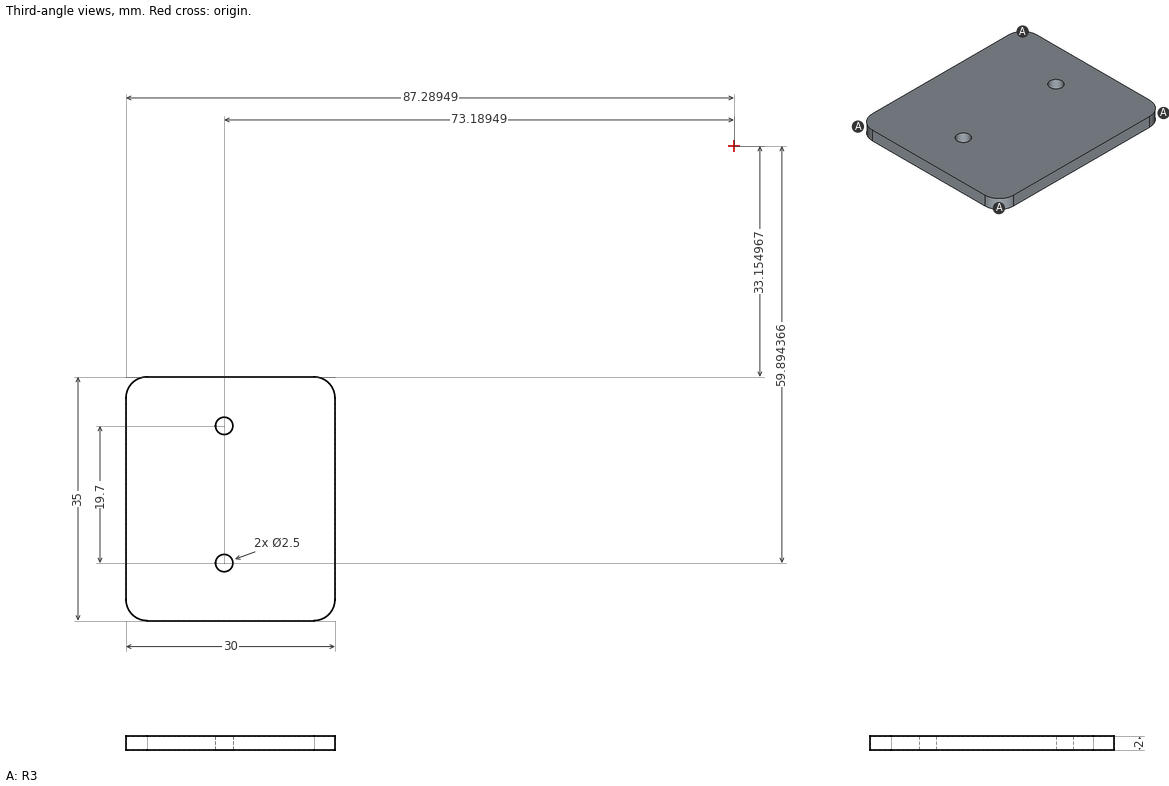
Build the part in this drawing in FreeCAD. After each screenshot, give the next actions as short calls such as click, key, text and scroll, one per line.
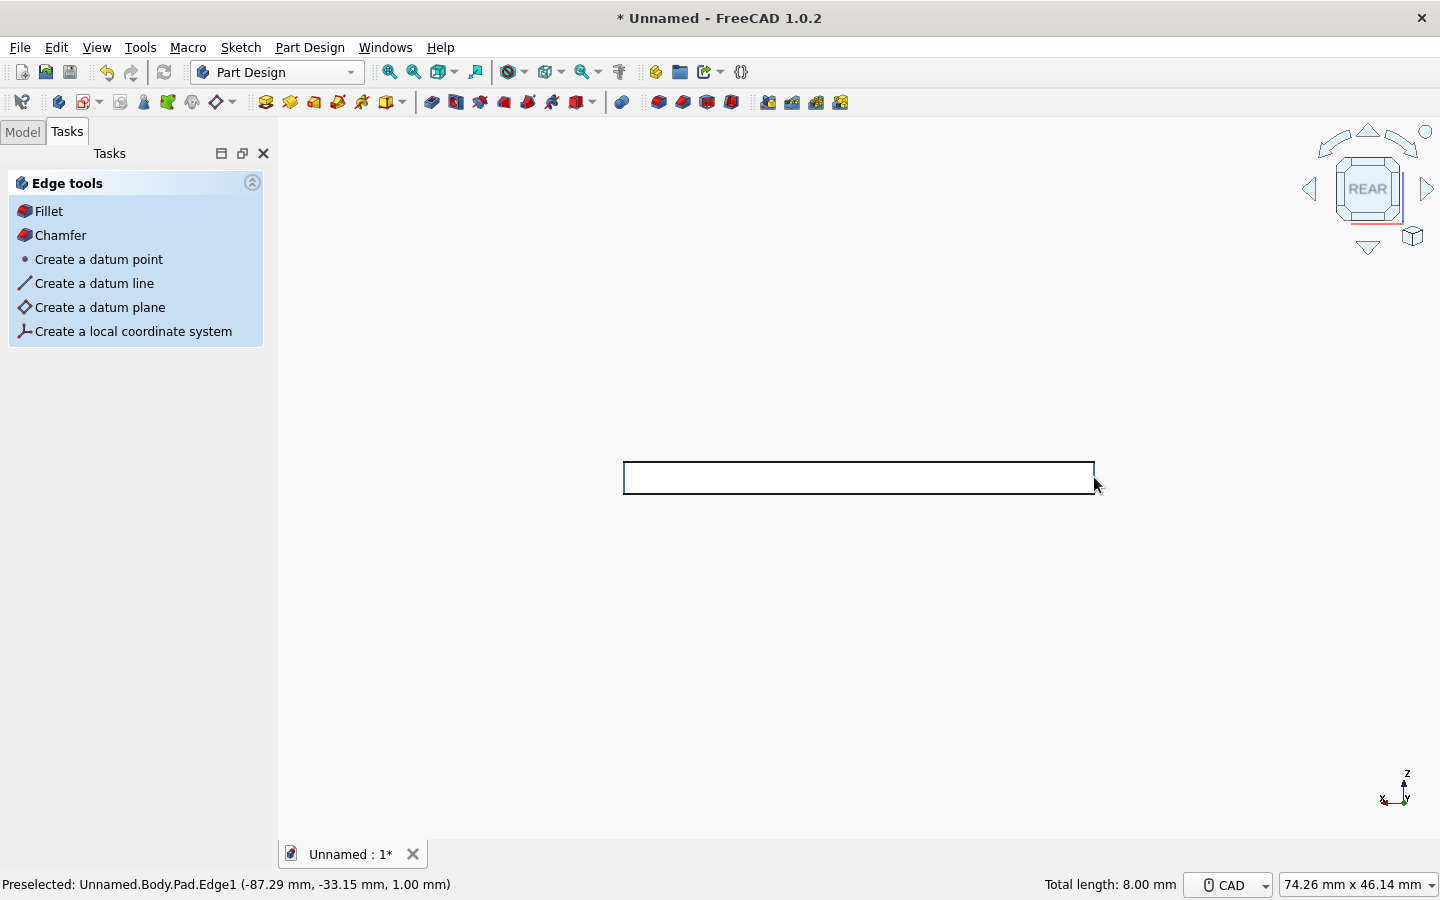
click(660, 102)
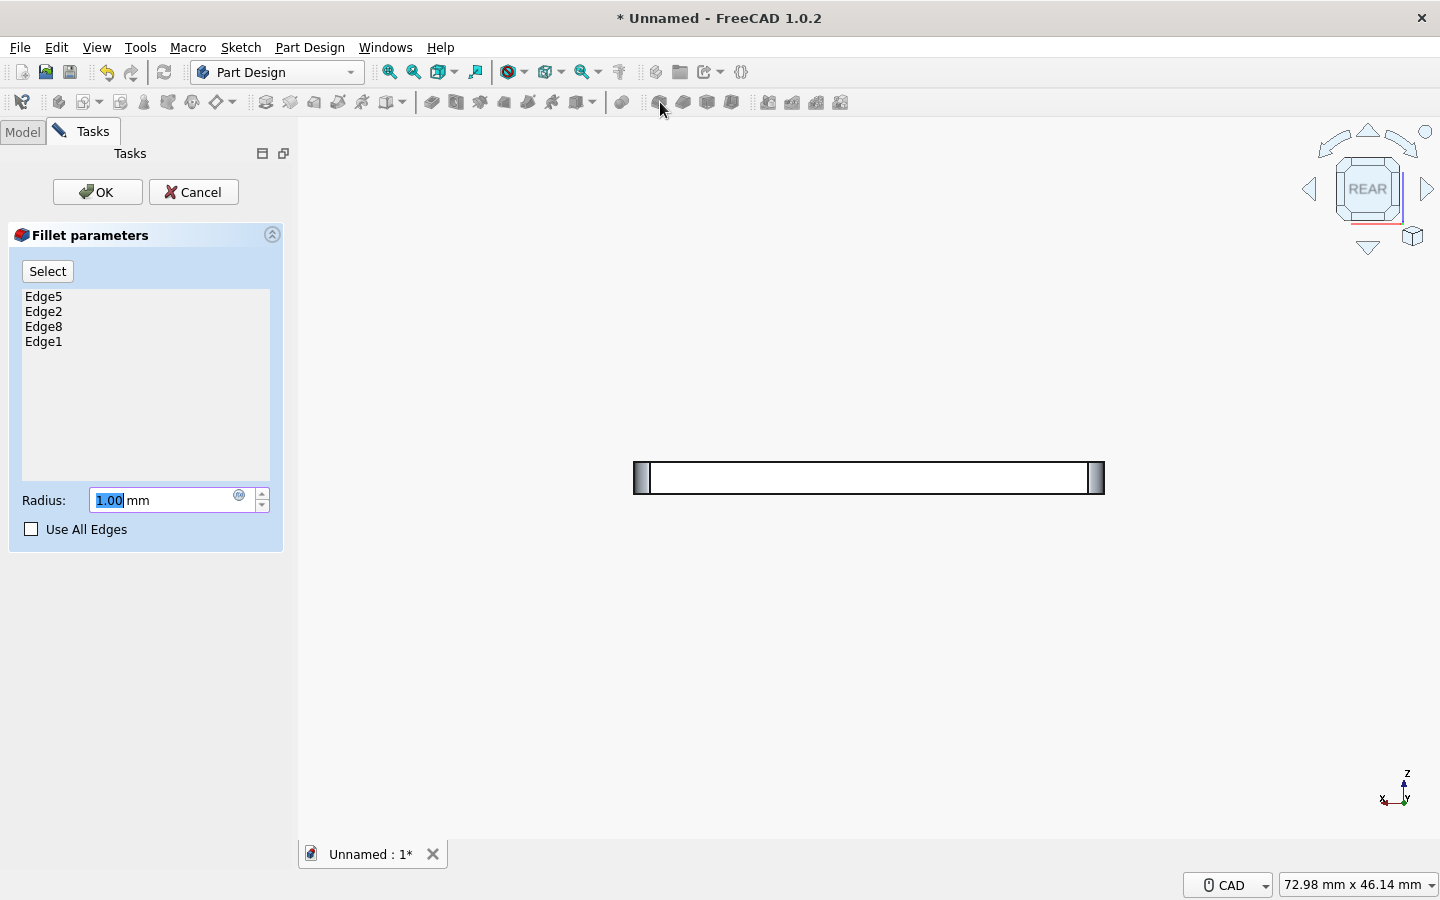
text(3)
key(Tab)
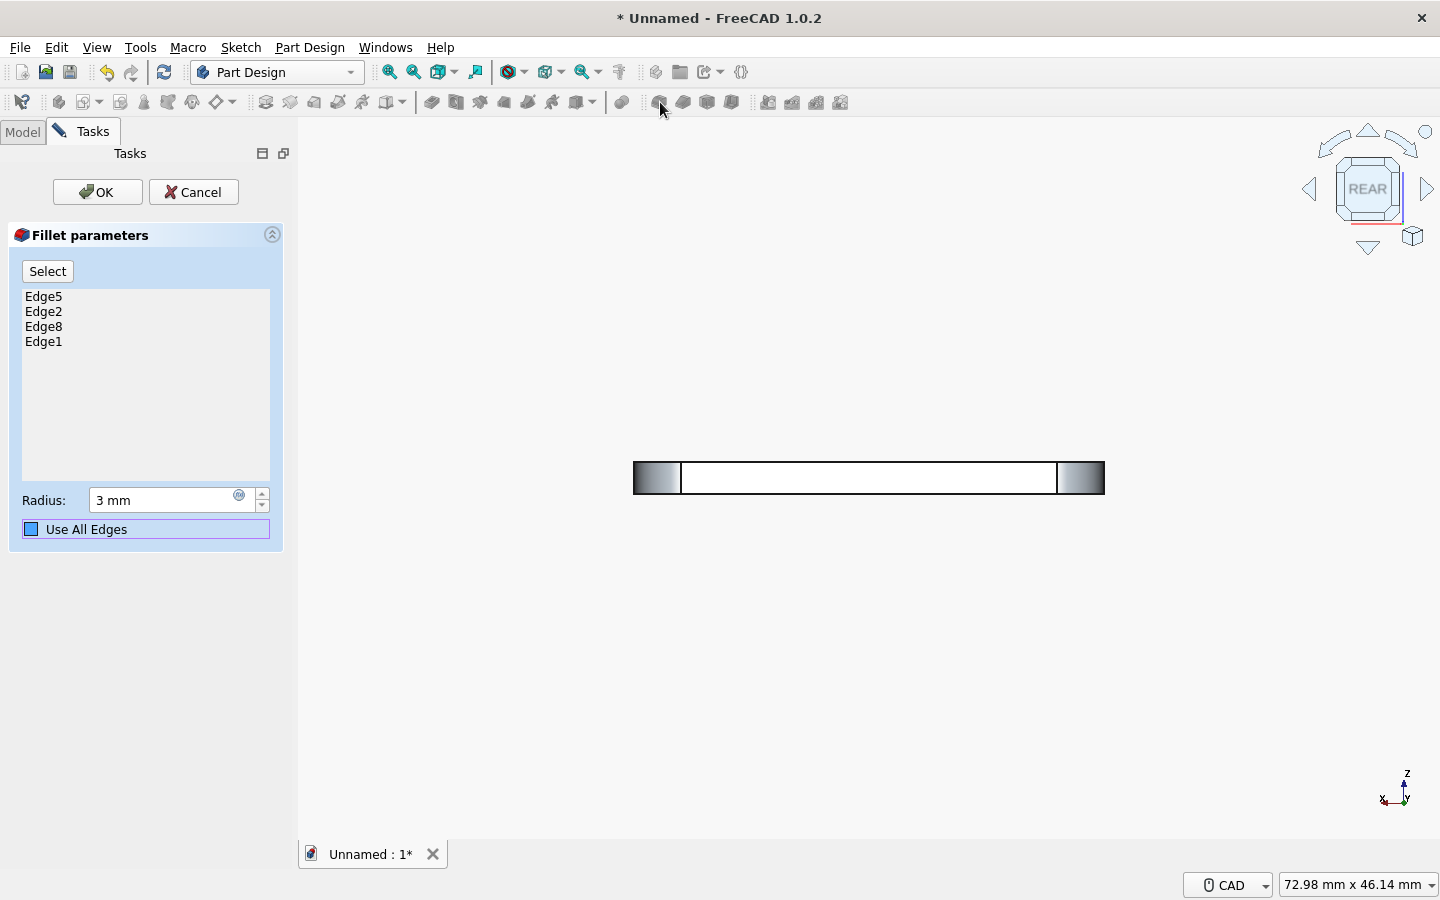
click(98, 192)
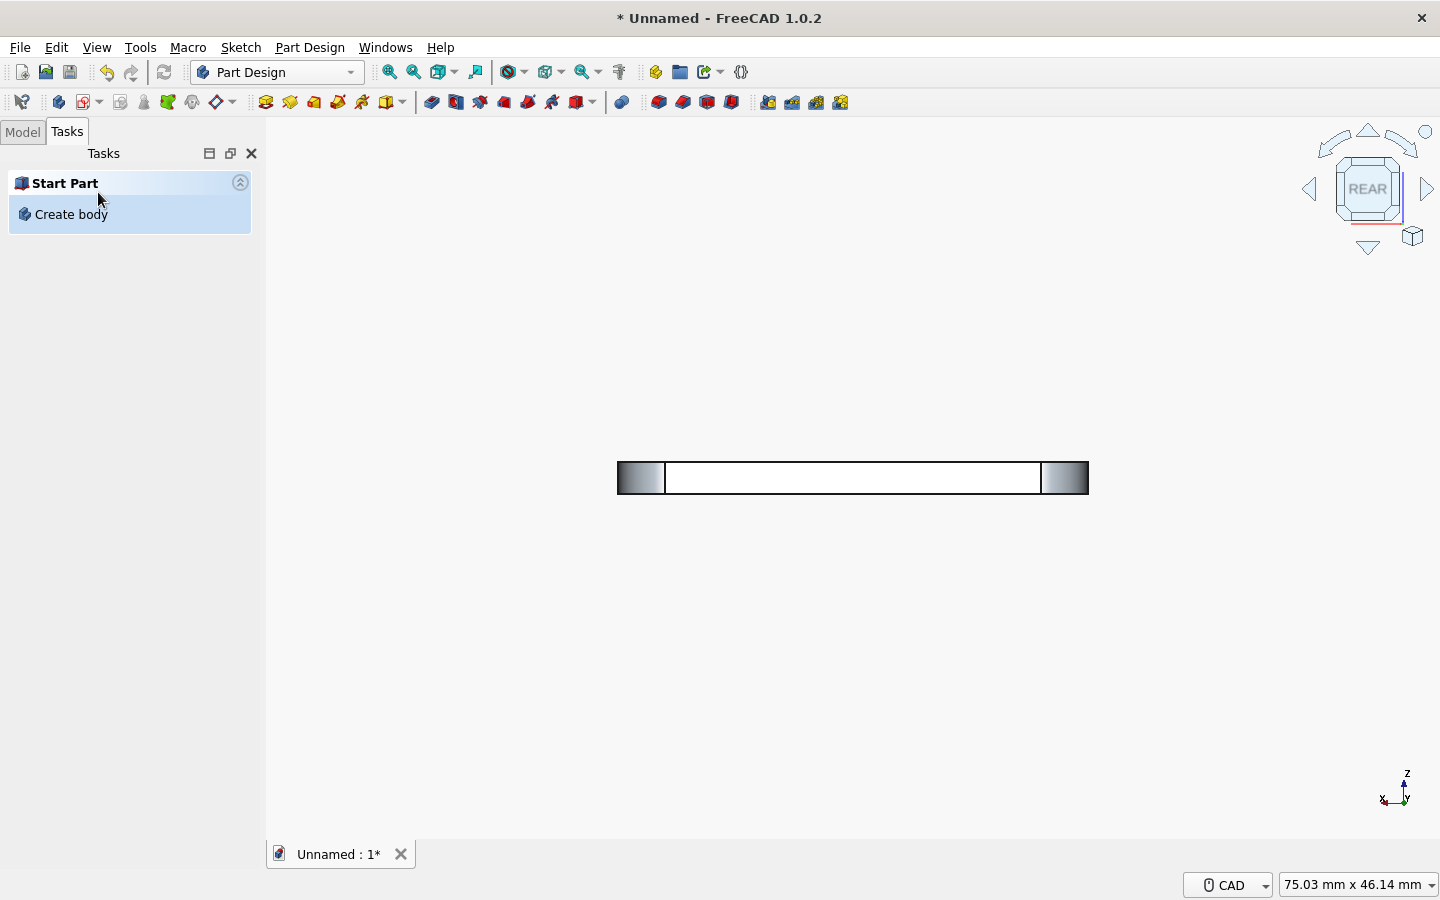
click(390, 72)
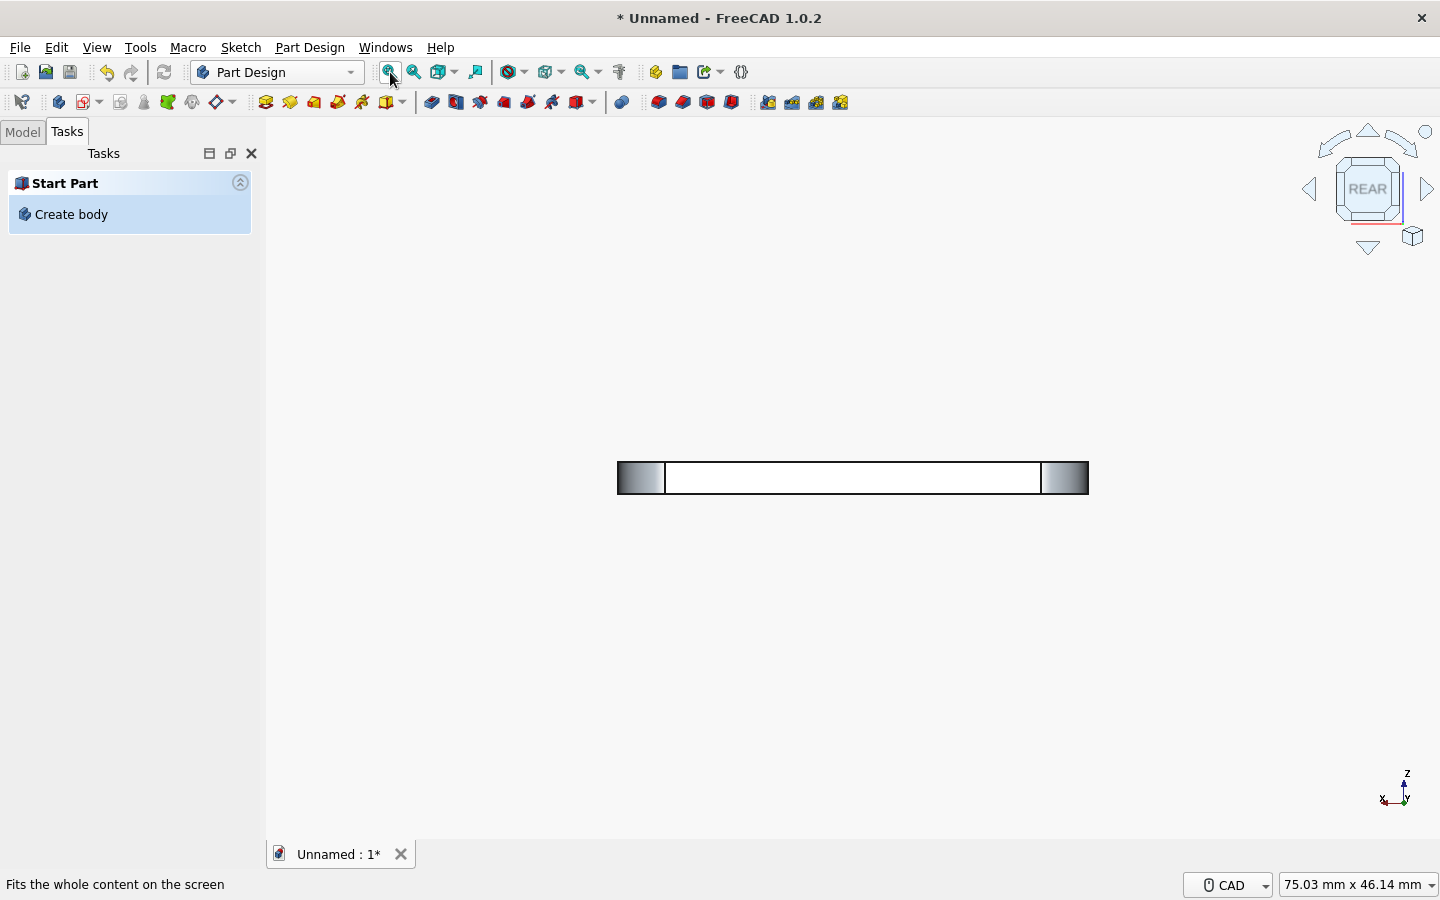
key(0)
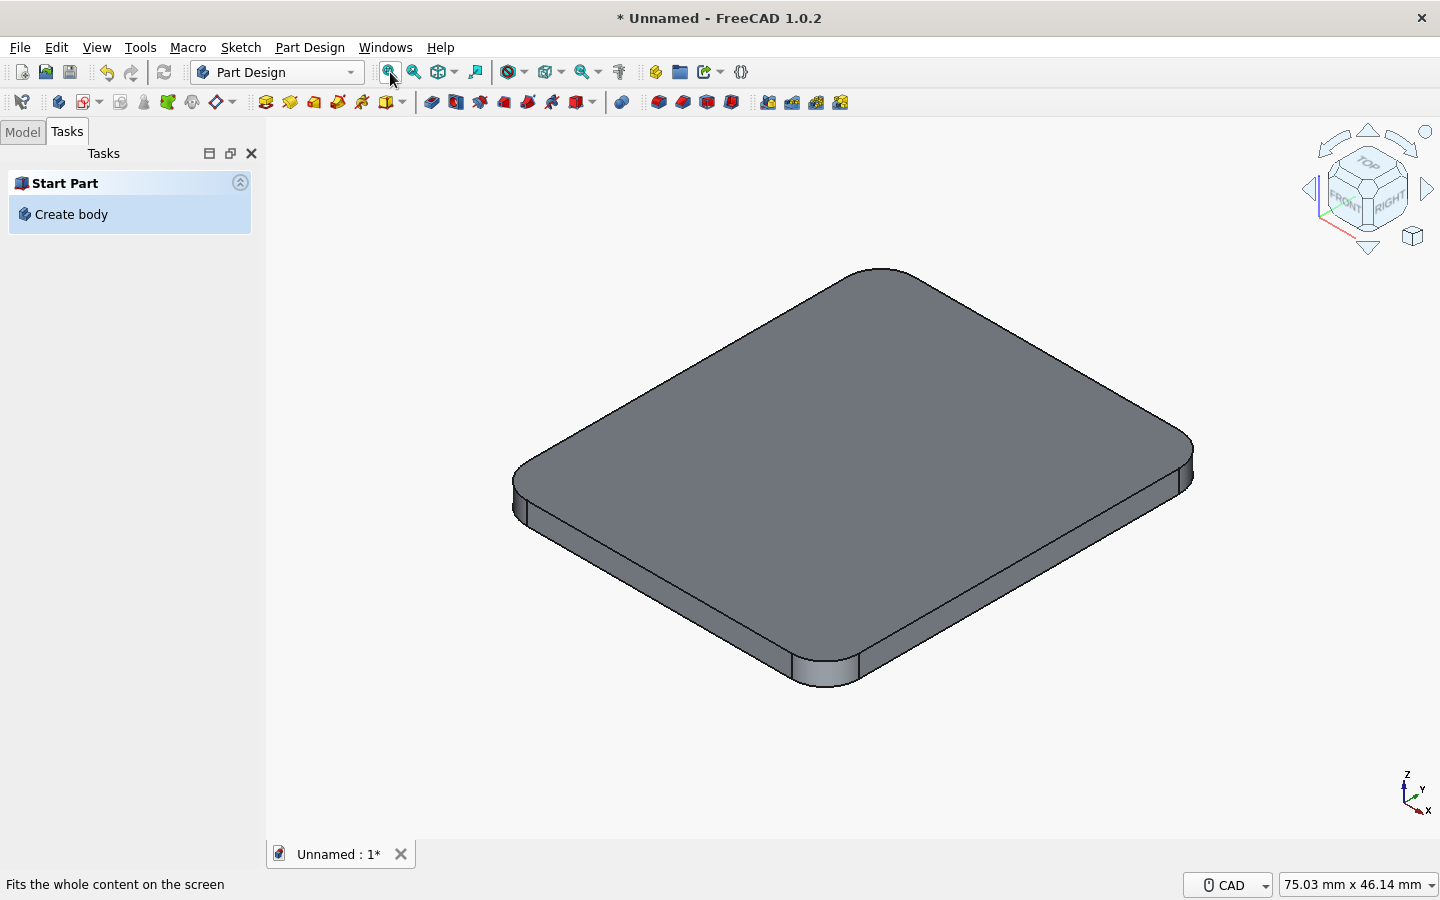
click(853, 464)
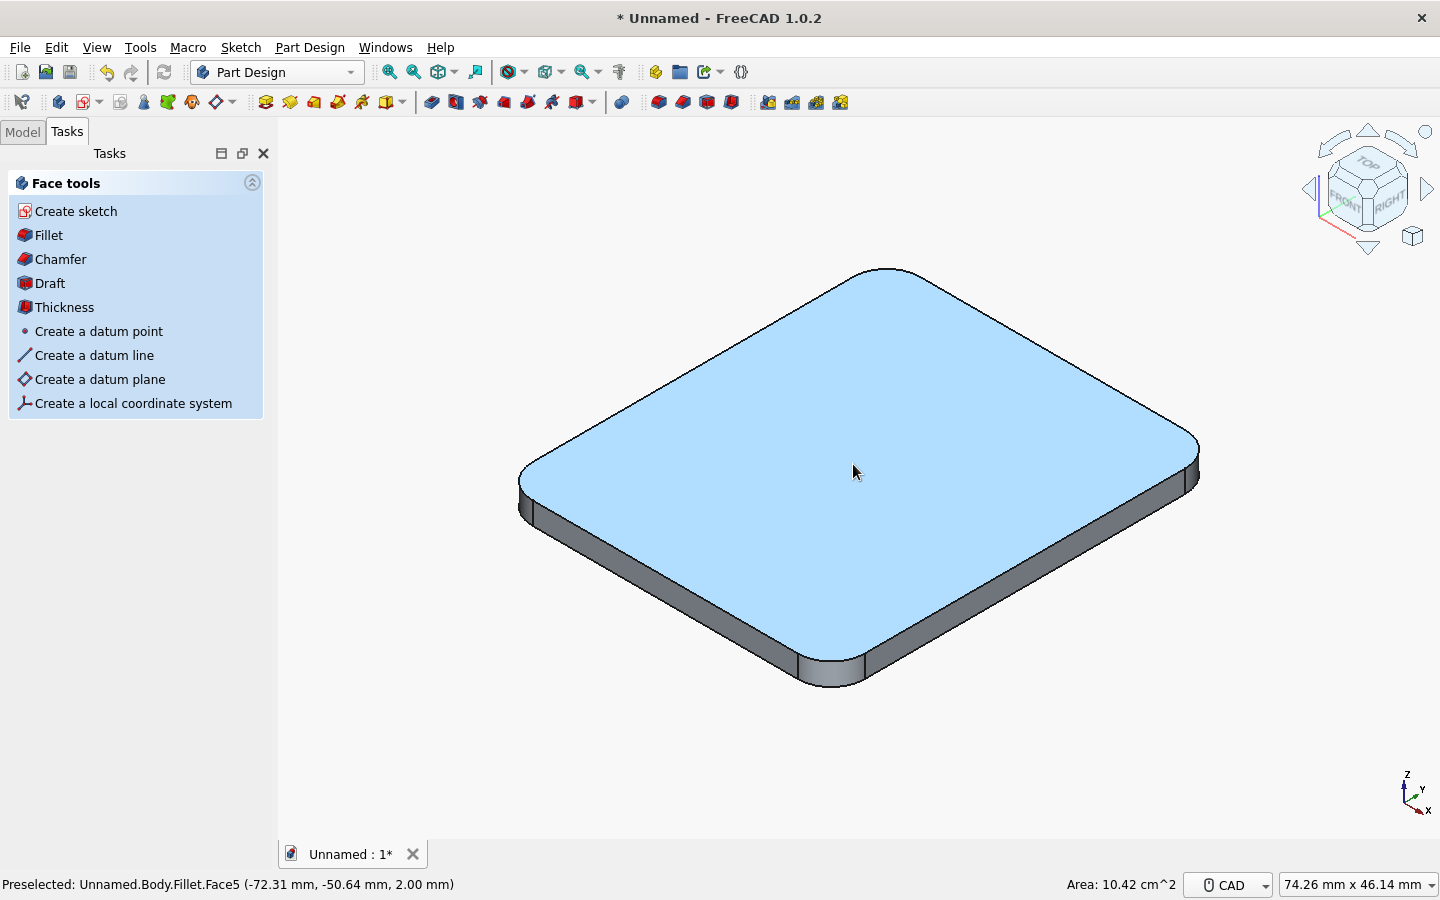
click(84, 102)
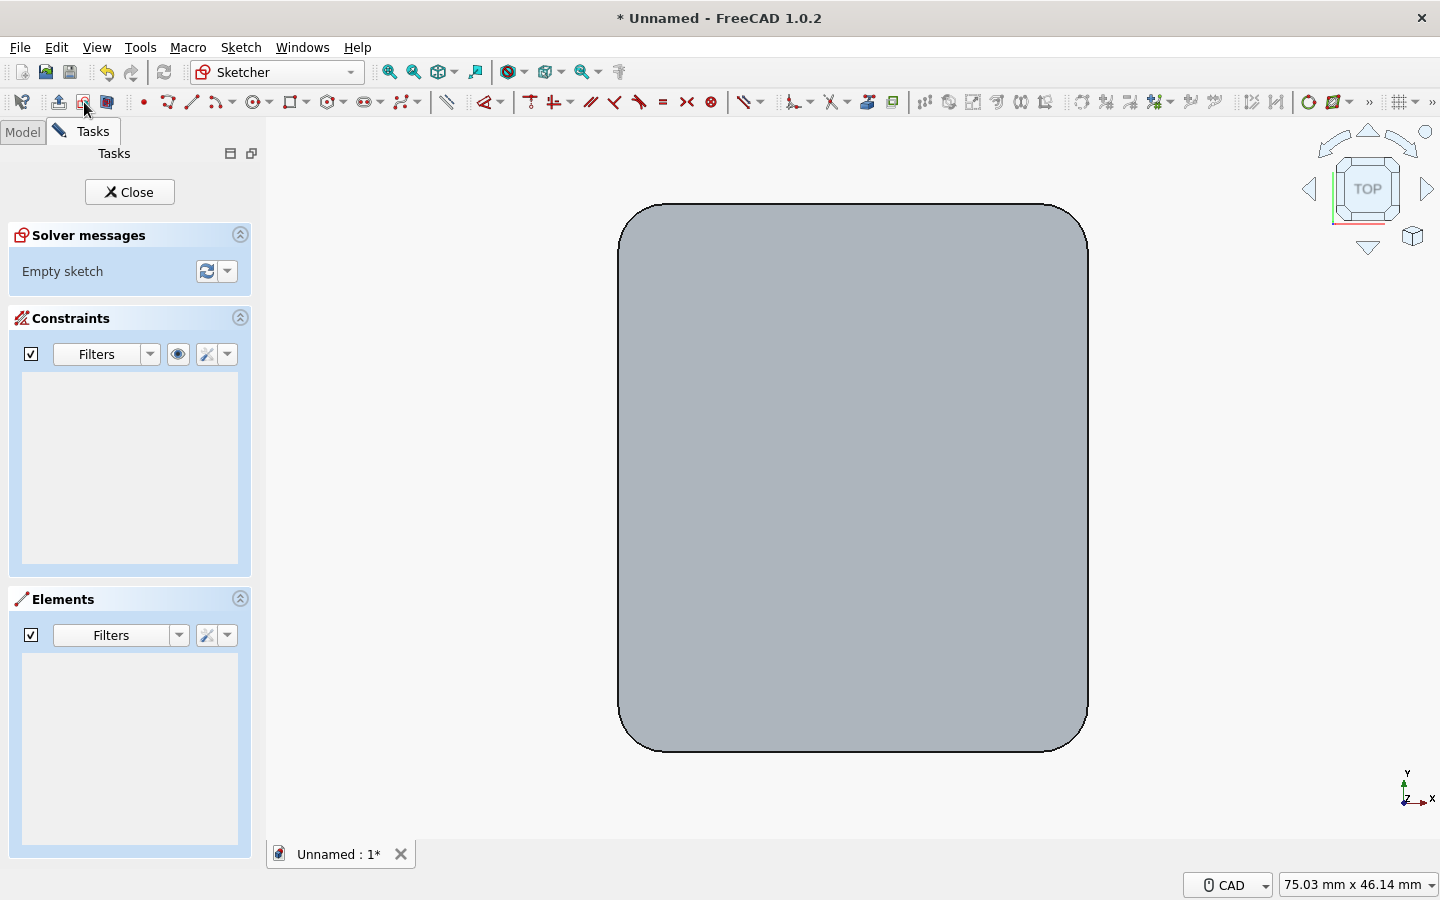
scroll(950, 449, up, 2)